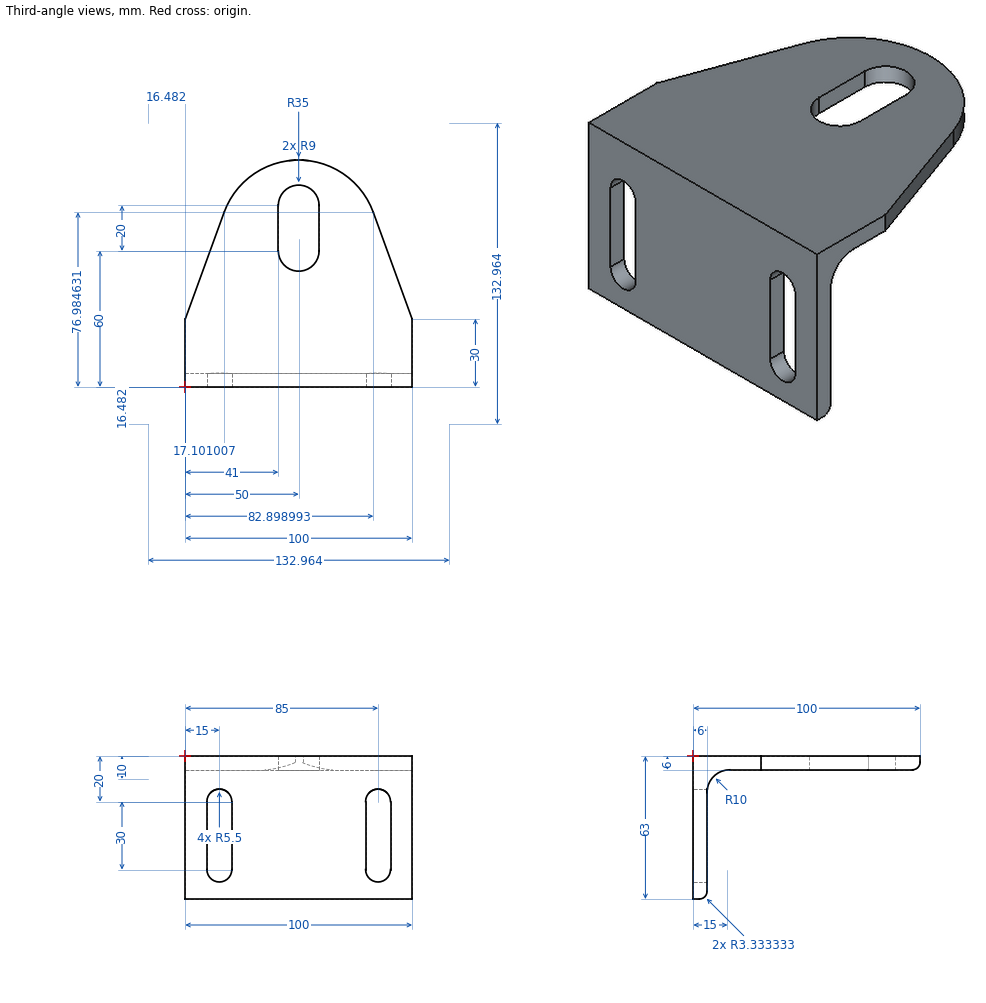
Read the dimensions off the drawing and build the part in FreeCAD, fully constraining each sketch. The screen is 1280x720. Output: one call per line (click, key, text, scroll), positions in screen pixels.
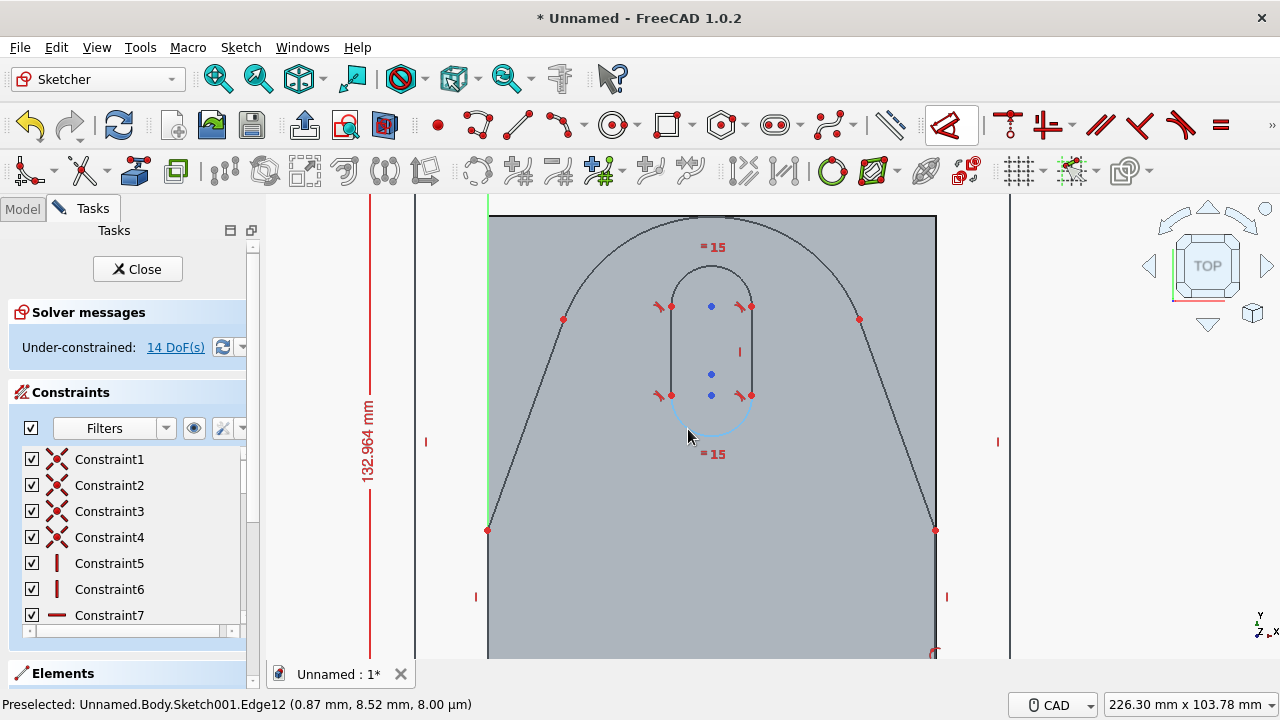
click(688, 429)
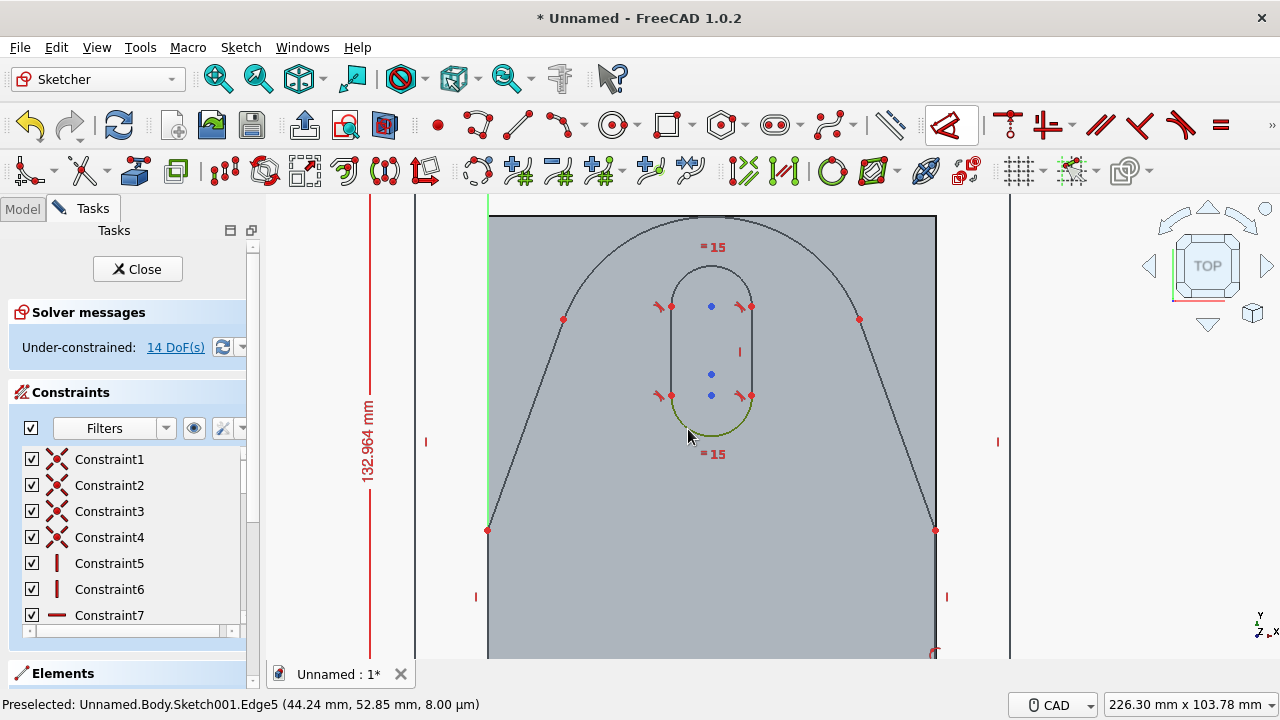
click(972, 126)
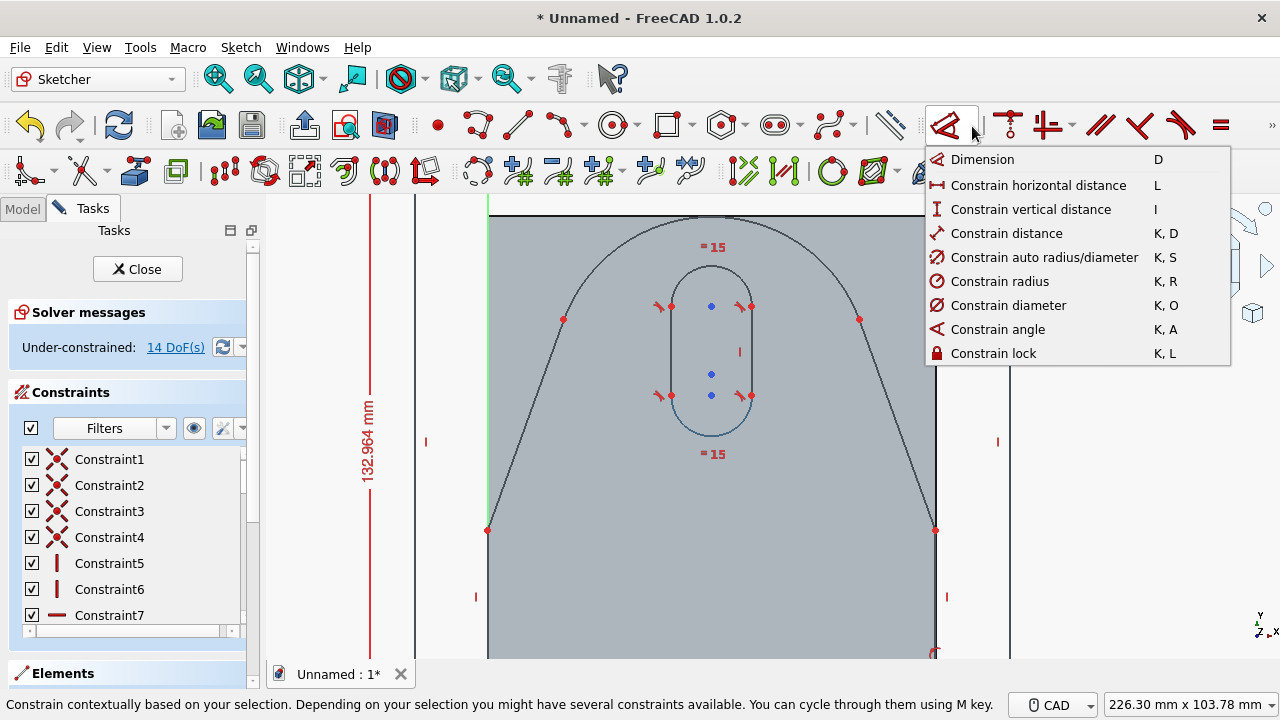
click(1078, 281)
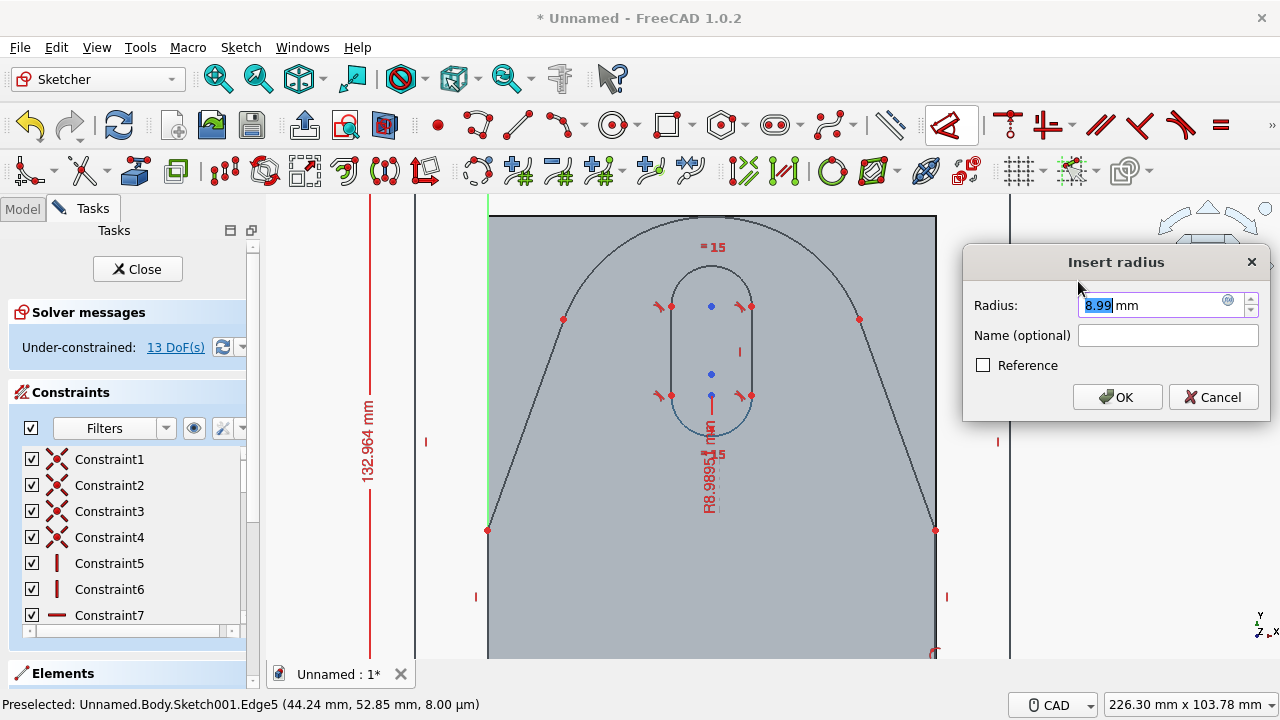
text(9)
key(Return)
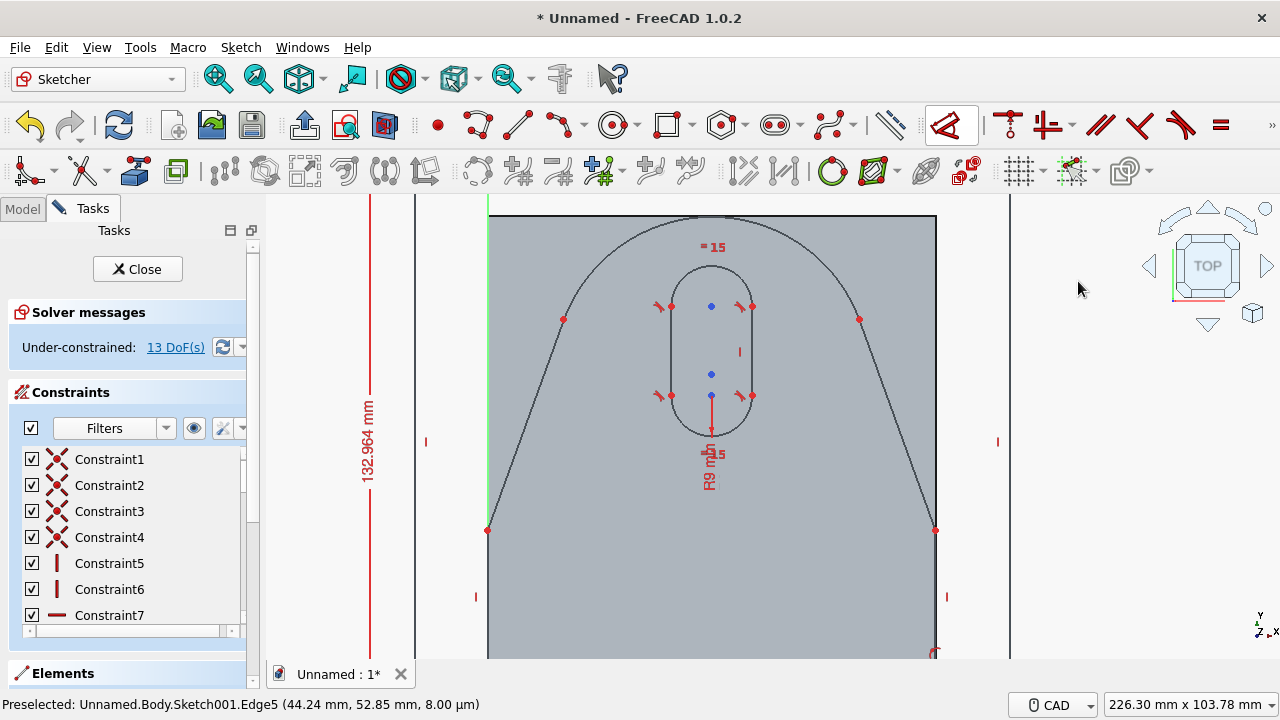
click(785, 235)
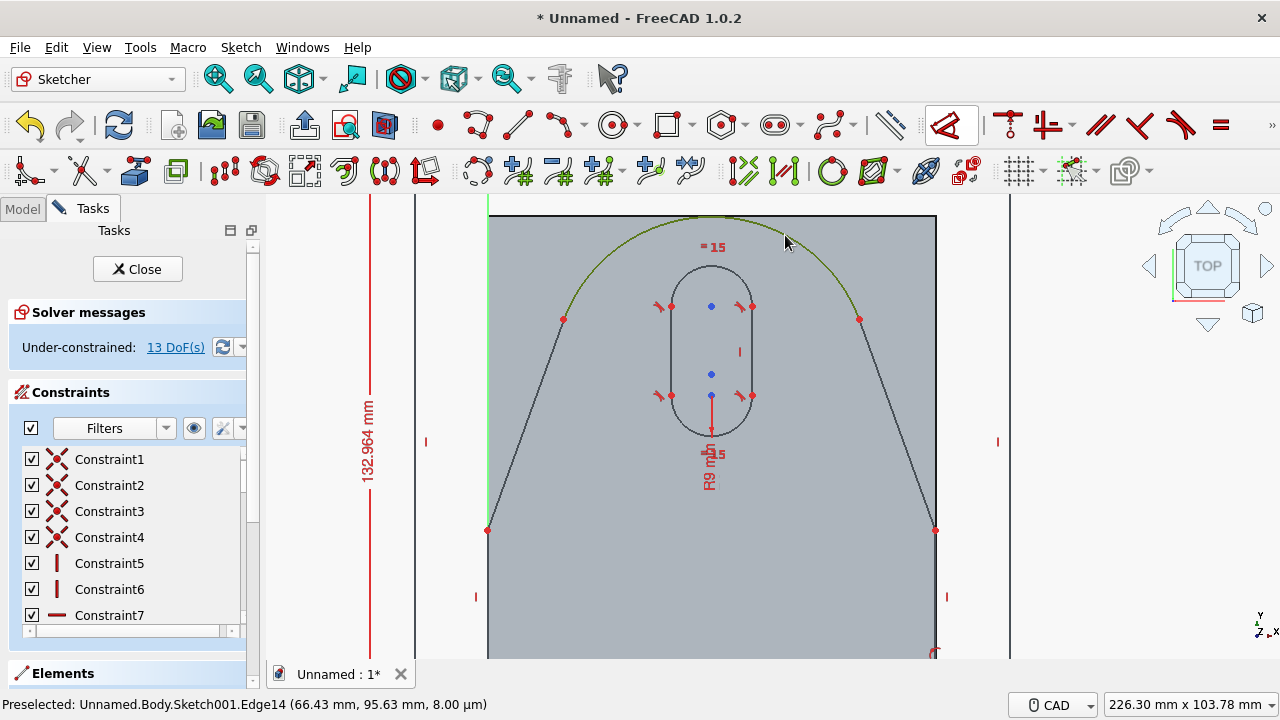
click(972, 126)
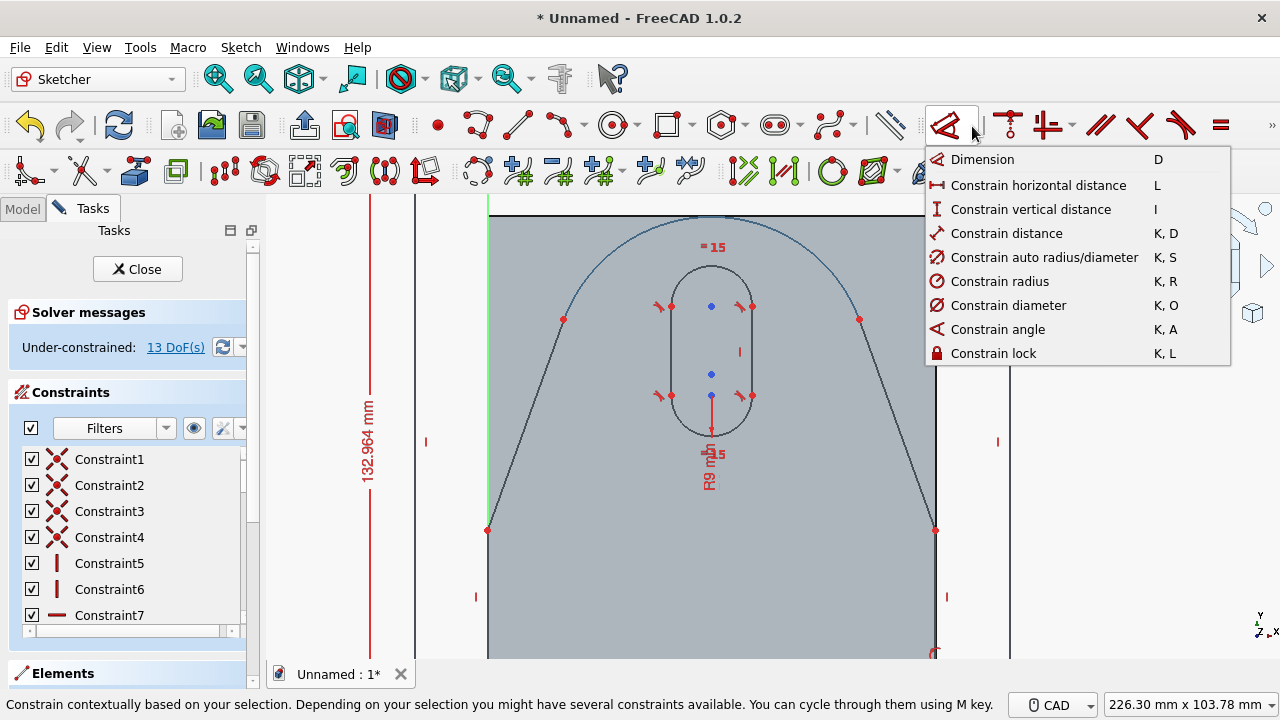
click(1078, 281)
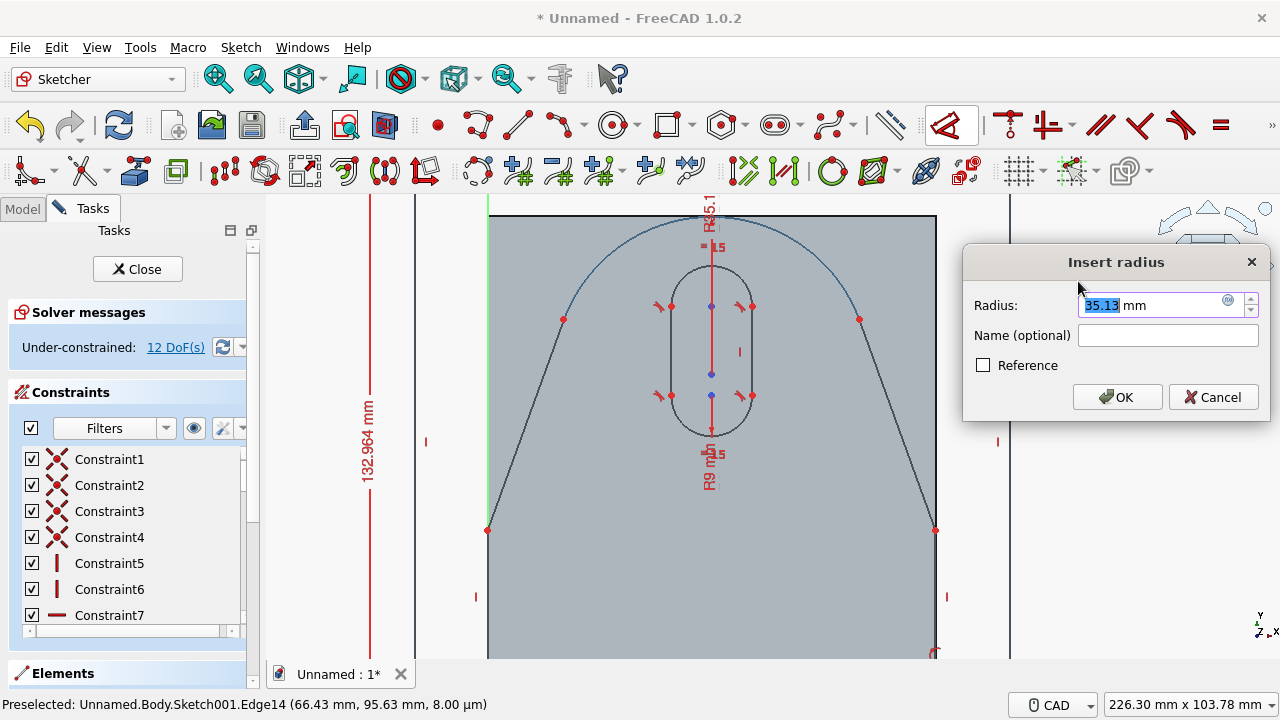
text(35)
key(Return)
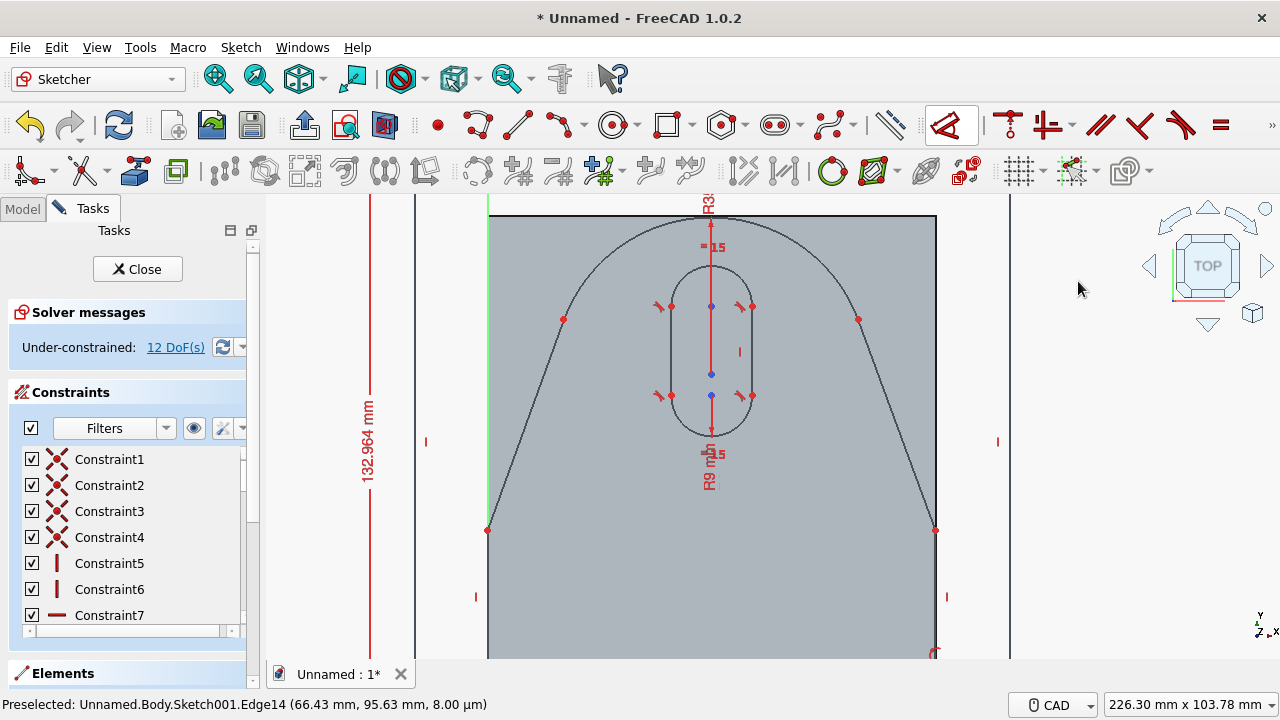
click(671, 369)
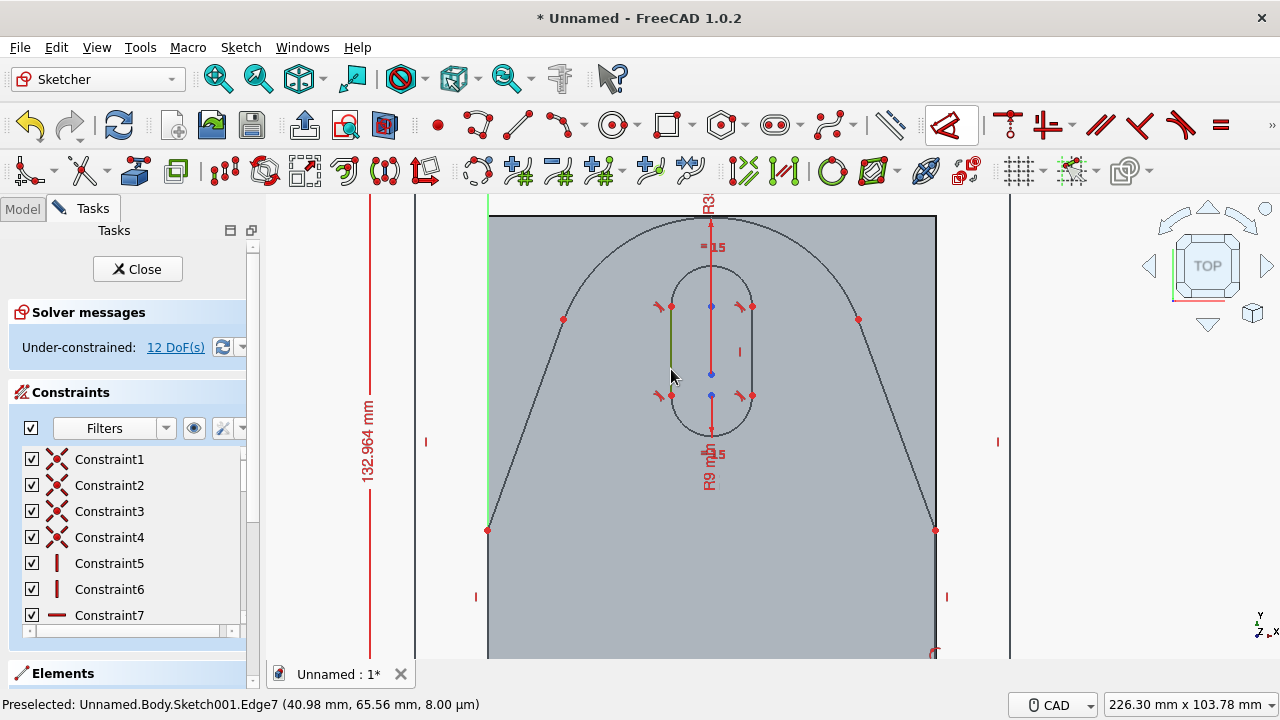
click(972, 126)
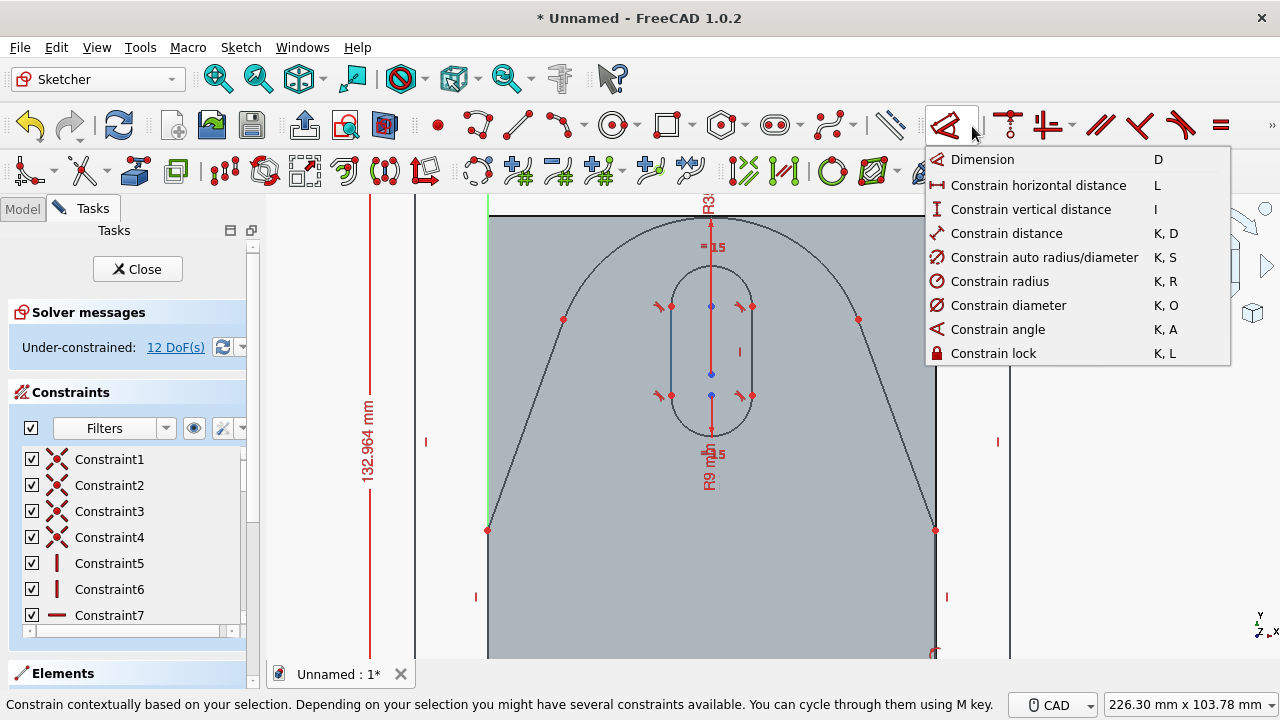
click(1078, 209)